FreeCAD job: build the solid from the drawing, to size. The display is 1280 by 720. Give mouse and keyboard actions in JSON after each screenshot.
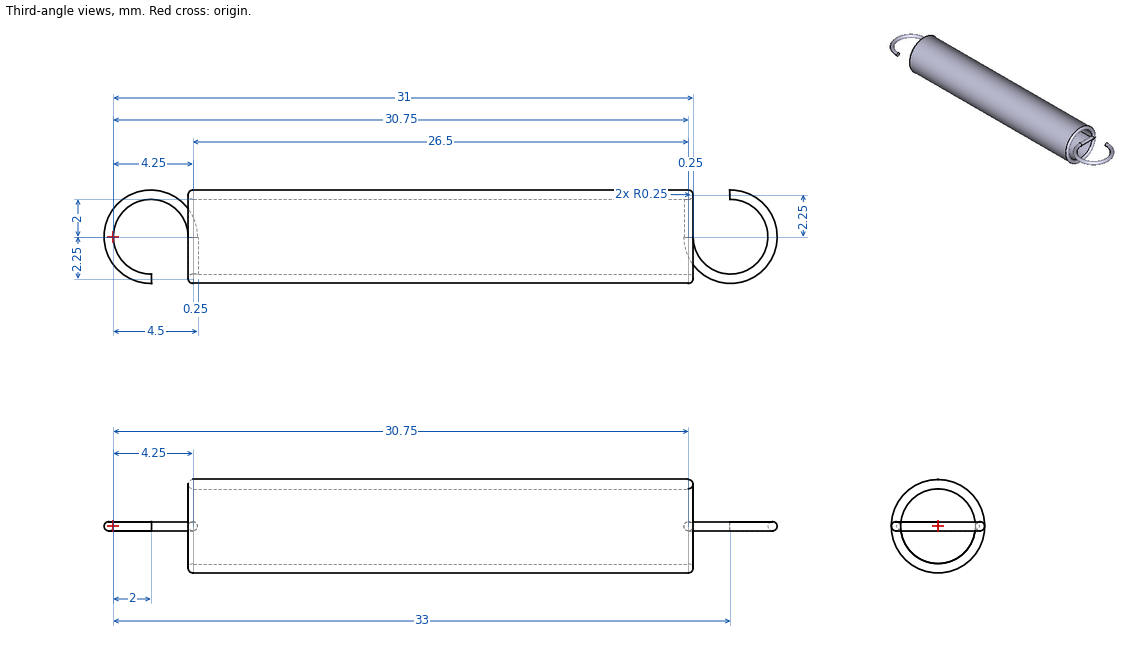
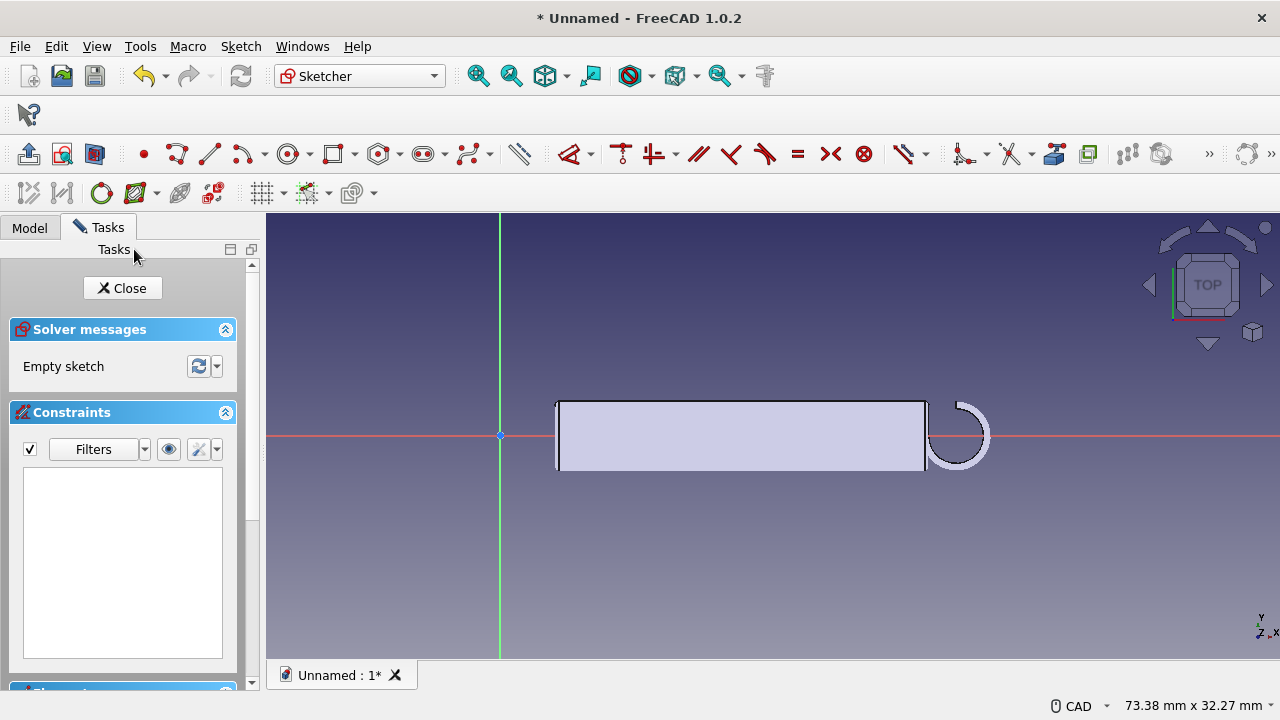
{"action": "key", "text": "q s"}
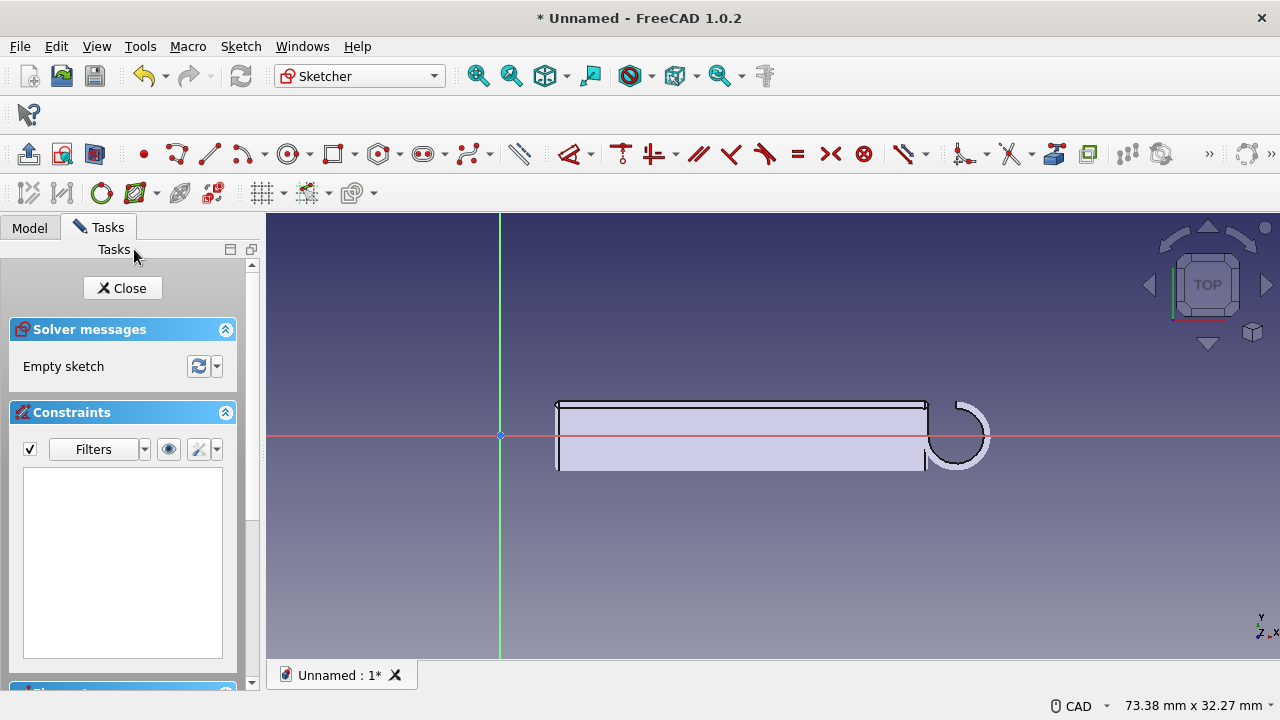
{"action": "scroll", "coordinate": [497, 447], "scroll_direction": "up", "scroll_amount": 9}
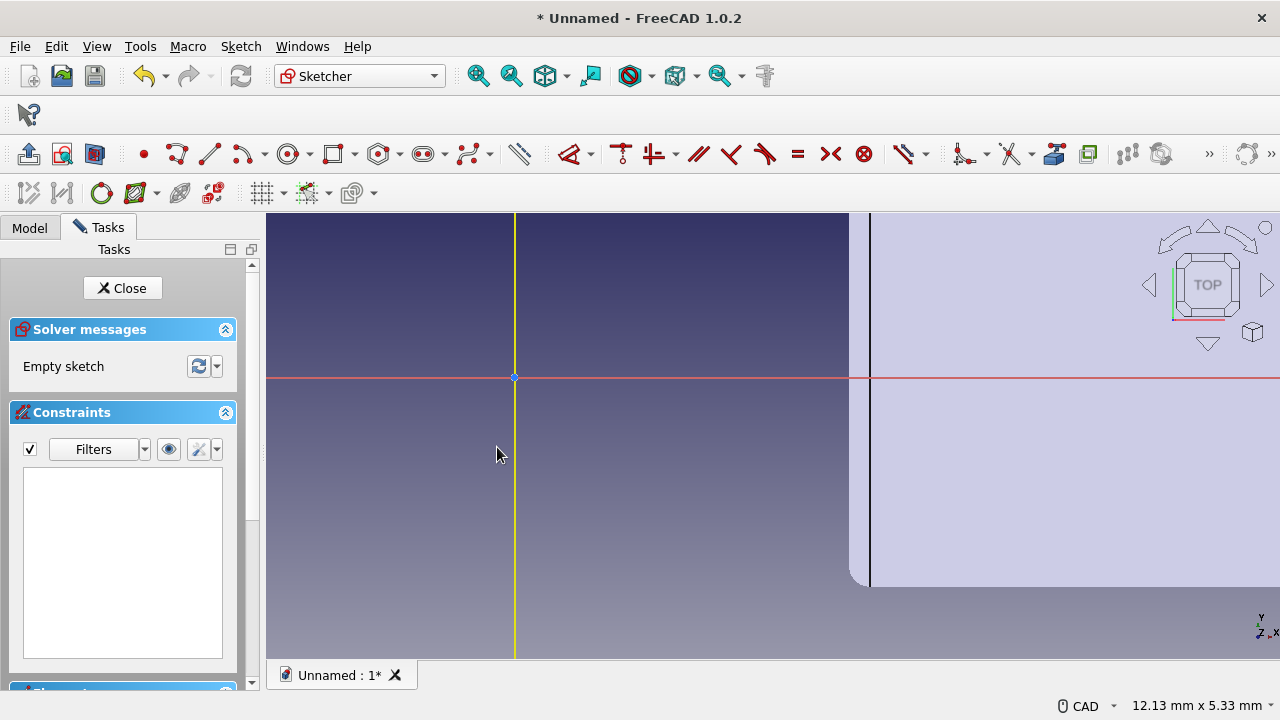
{"action": "key", "text": "g r"}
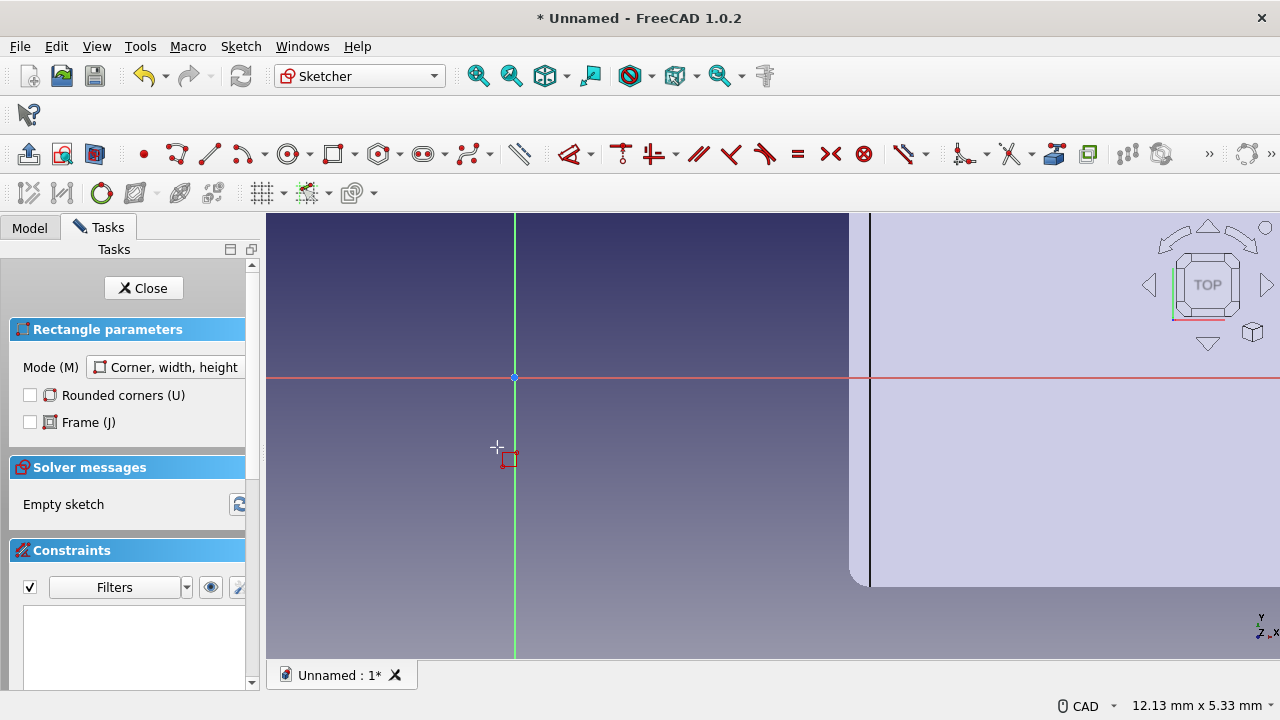
{"action": "left_click", "coordinate": [870, 378]}
{"action": "left_click", "coordinate": [891, 566]}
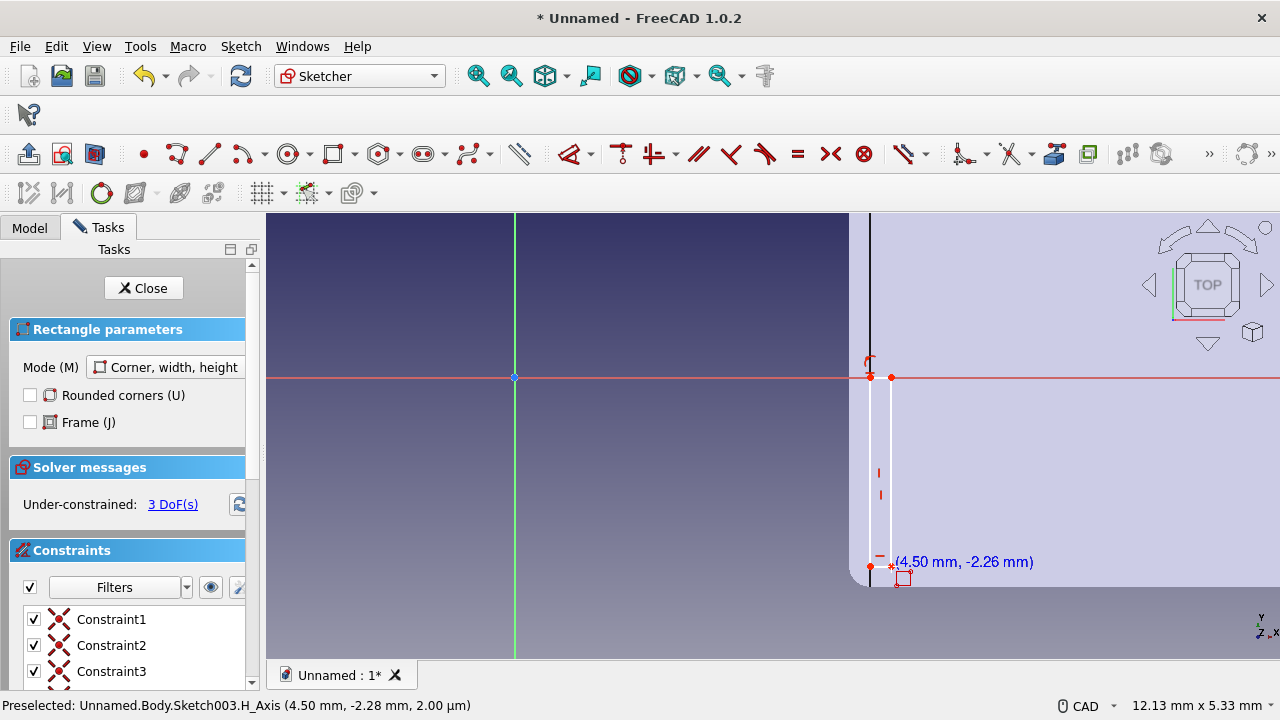
{"action": "key", "text": "g l"}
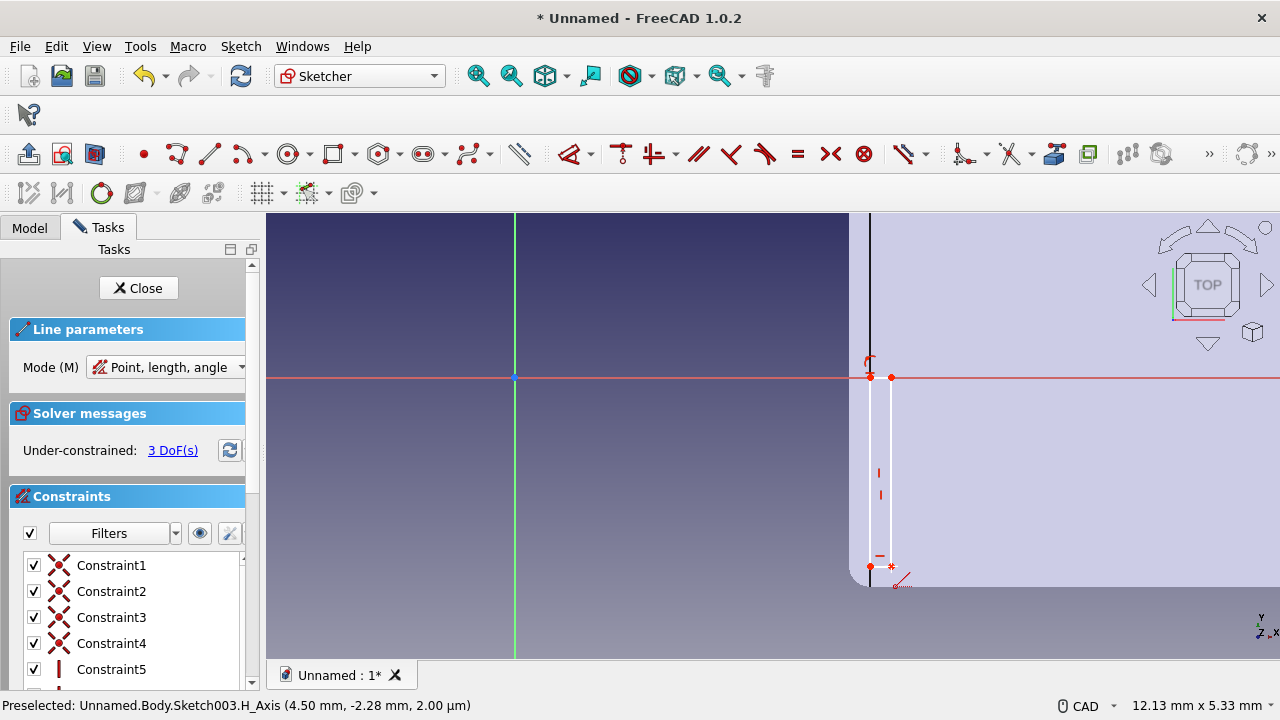
{"action": "left_click", "coordinate": [870, 359]}
{"action": "left_click", "coordinate": [870, 303]}
{"action": "key", "text": "Escape"}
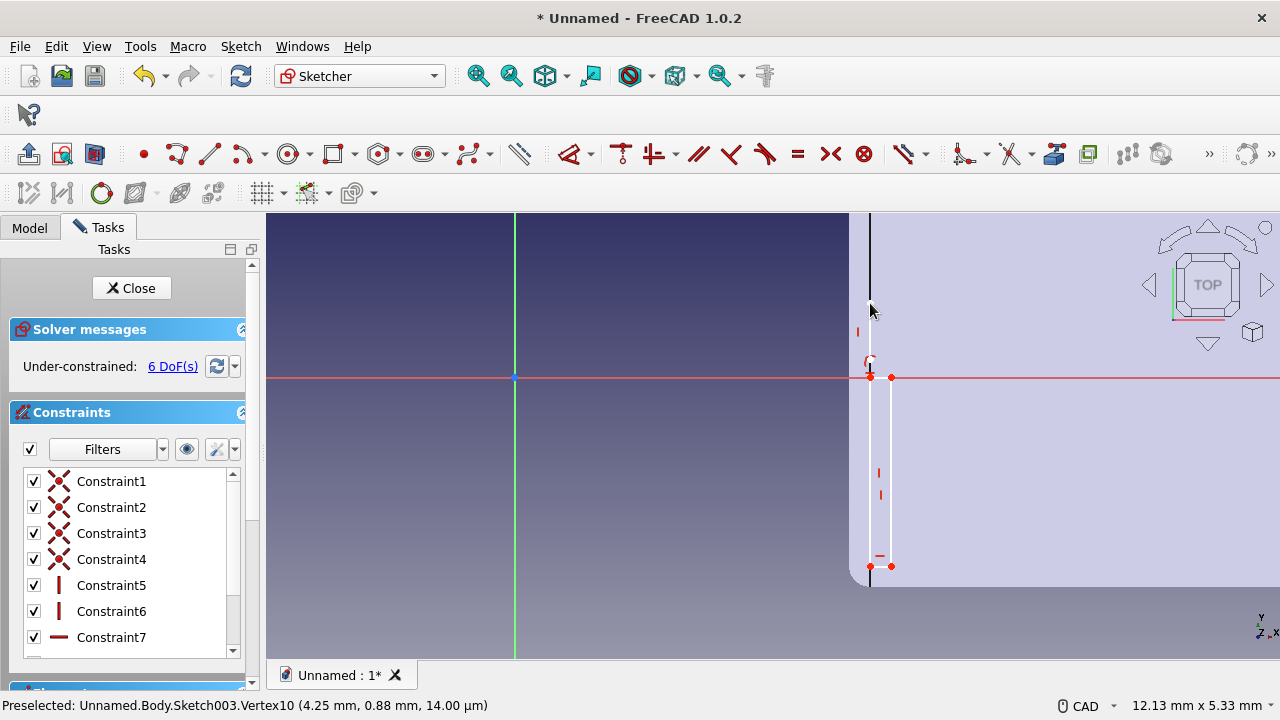
{"action": "left_click", "coordinate": [870, 343]}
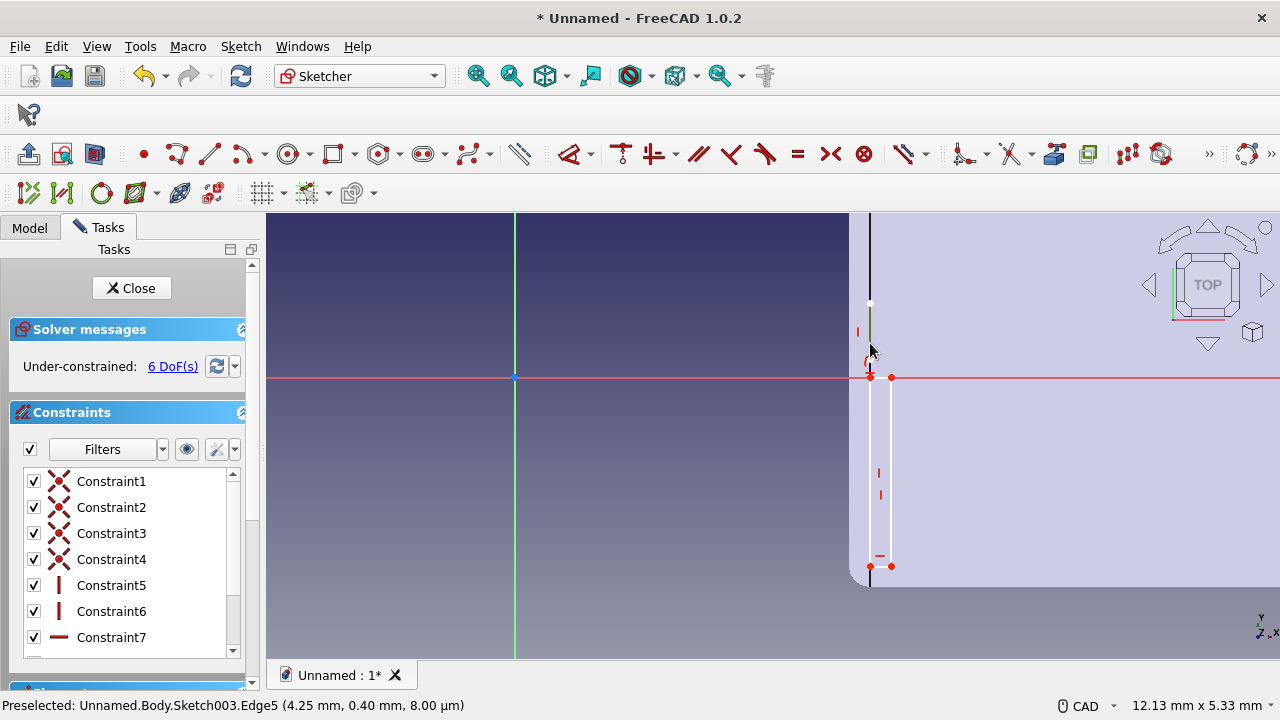
{"action": "key", "text": "g n"}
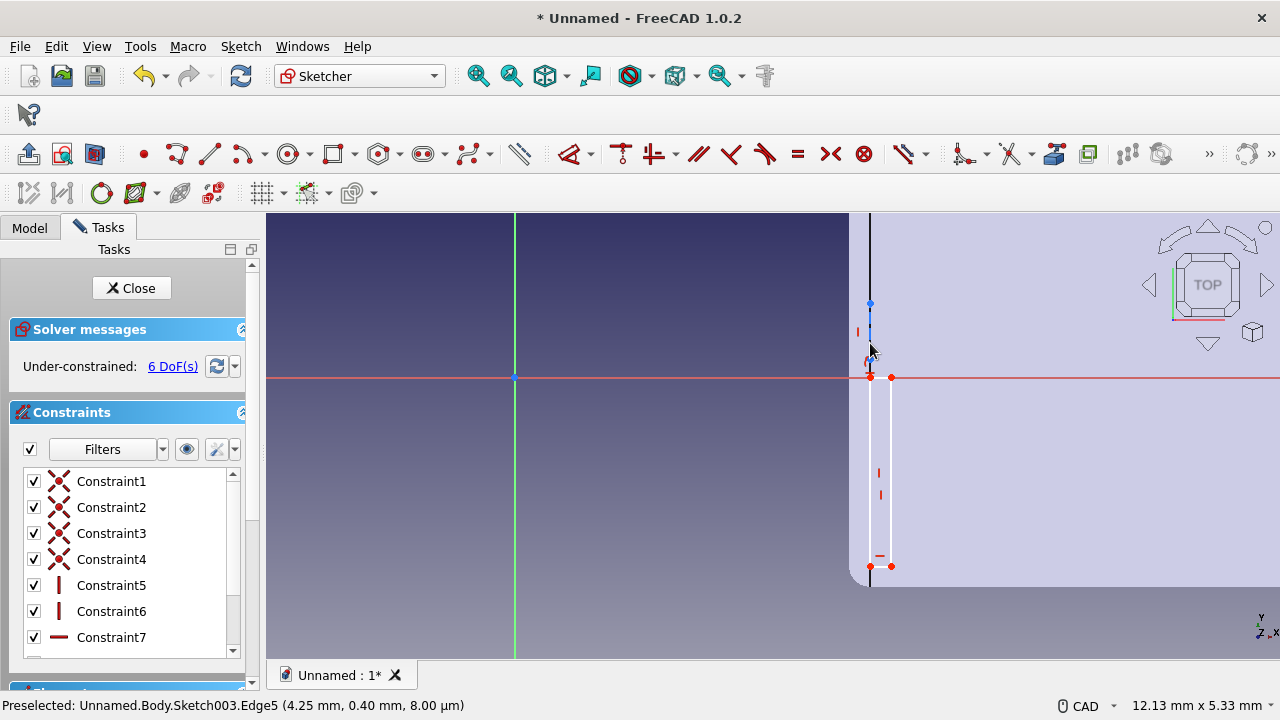
{"action": "left_click", "coordinate": [568, 154]}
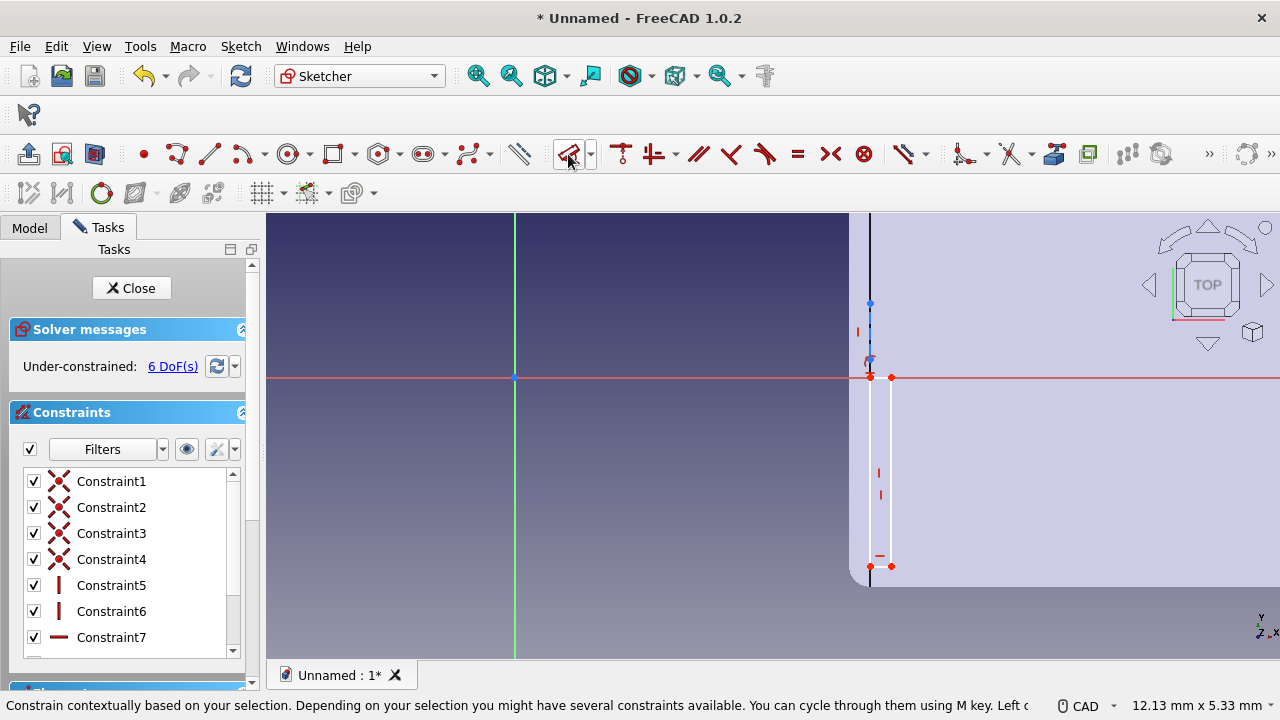
{"action": "left_click", "coordinate": [870, 435]}
{"action": "left_click", "coordinate": [836, 472]}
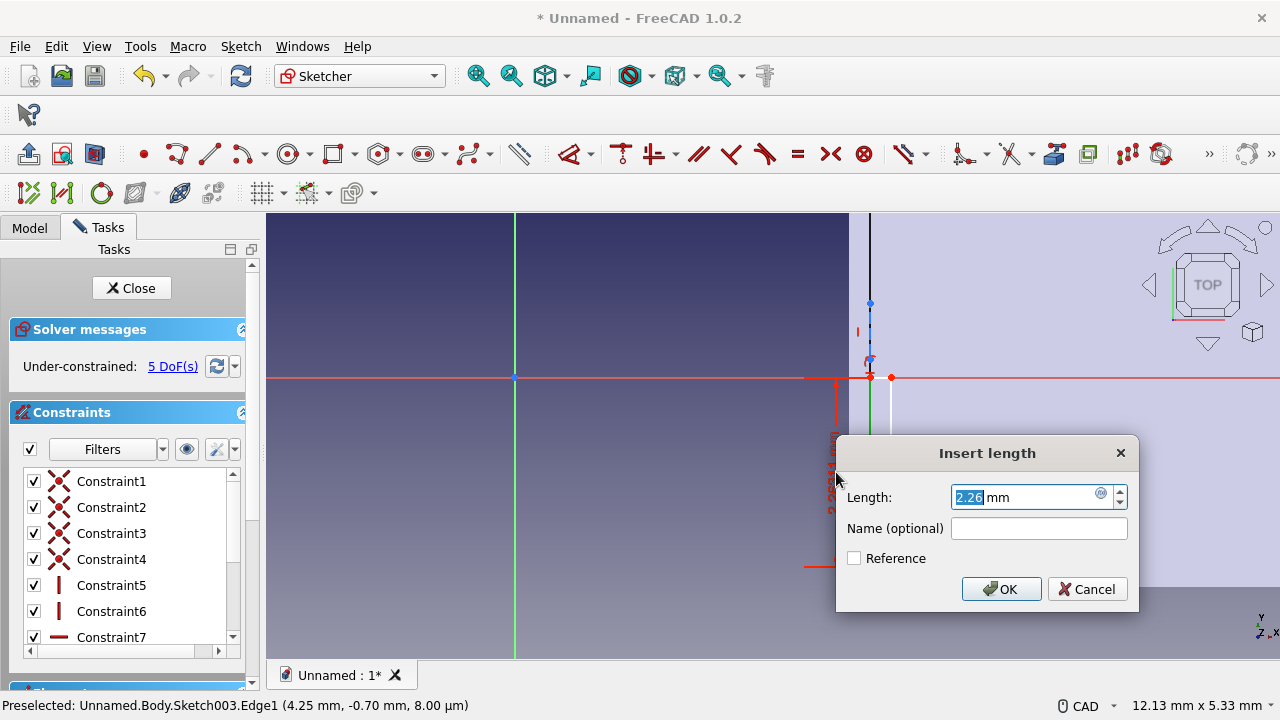
{"action": "type", "text": "2.25"}
{"action": "key", "text": "Return"}